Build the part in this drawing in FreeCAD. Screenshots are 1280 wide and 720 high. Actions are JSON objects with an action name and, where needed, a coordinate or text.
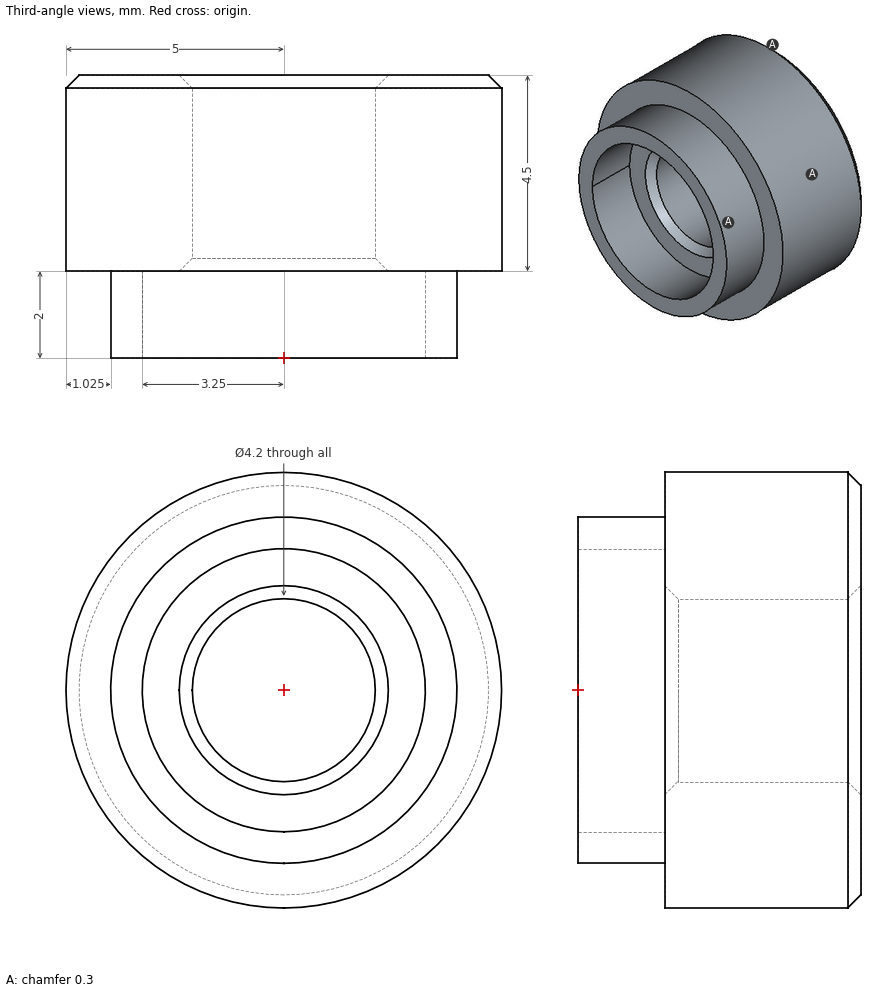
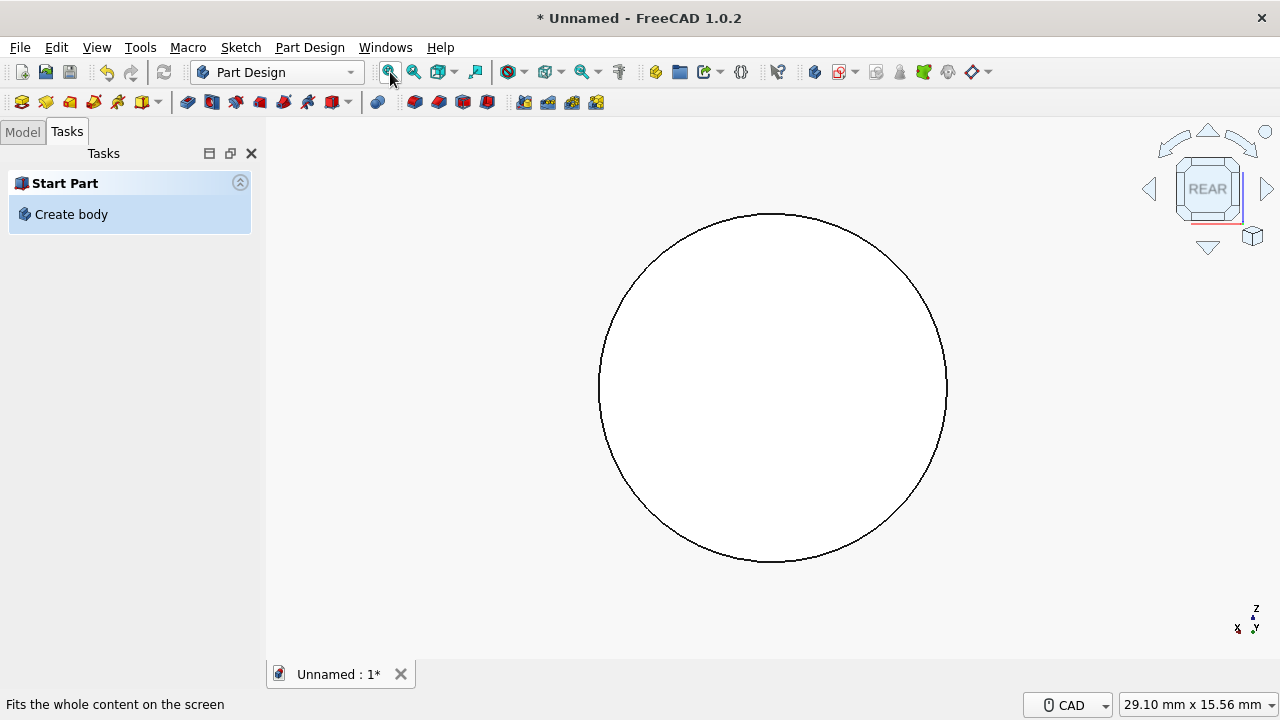
{"action": "left_click", "coordinate": [773, 387]}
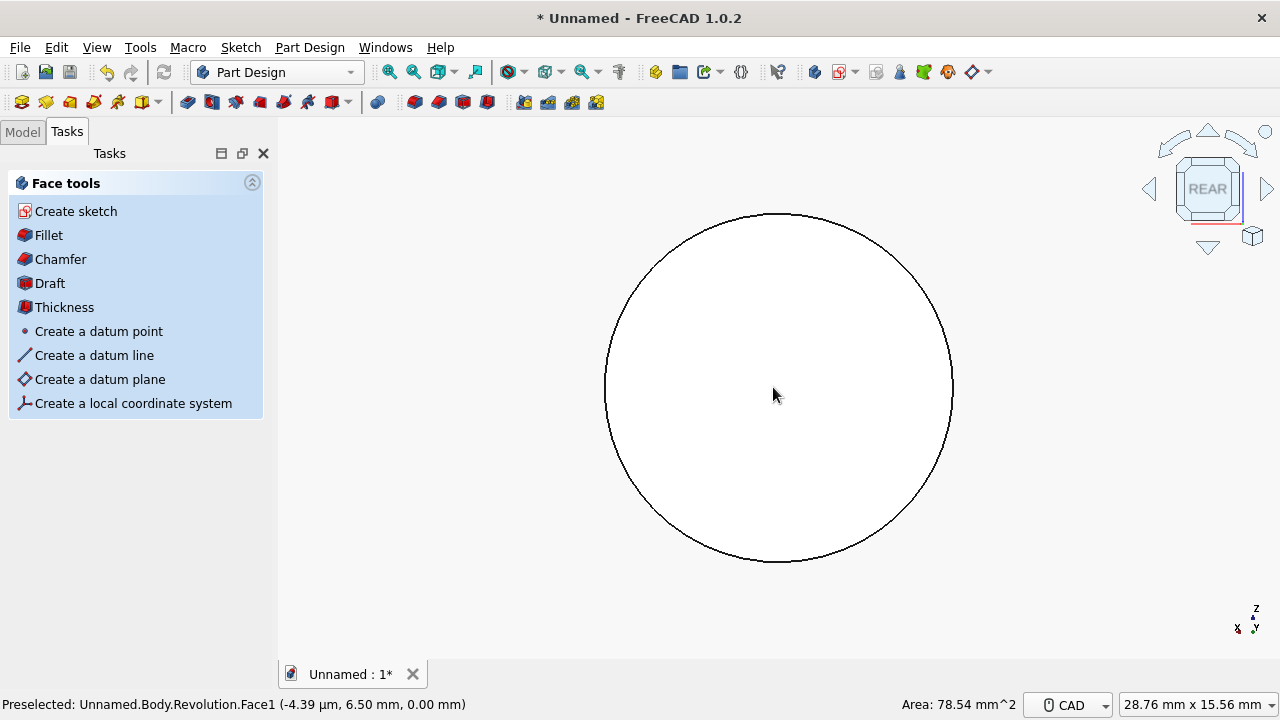
{"action": "left_click", "coordinate": [840, 72]}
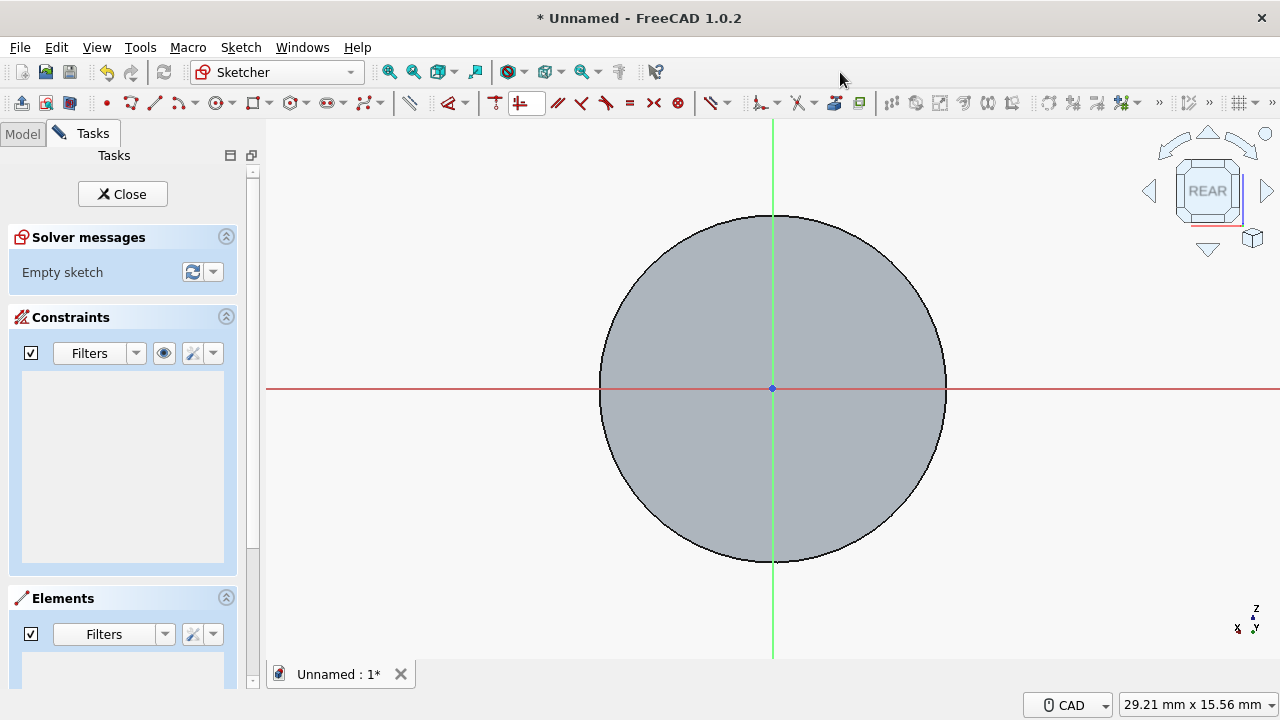
{"action": "scroll", "coordinate": [829, 389], "scroll_direction": "up", "scroll_amount": 4}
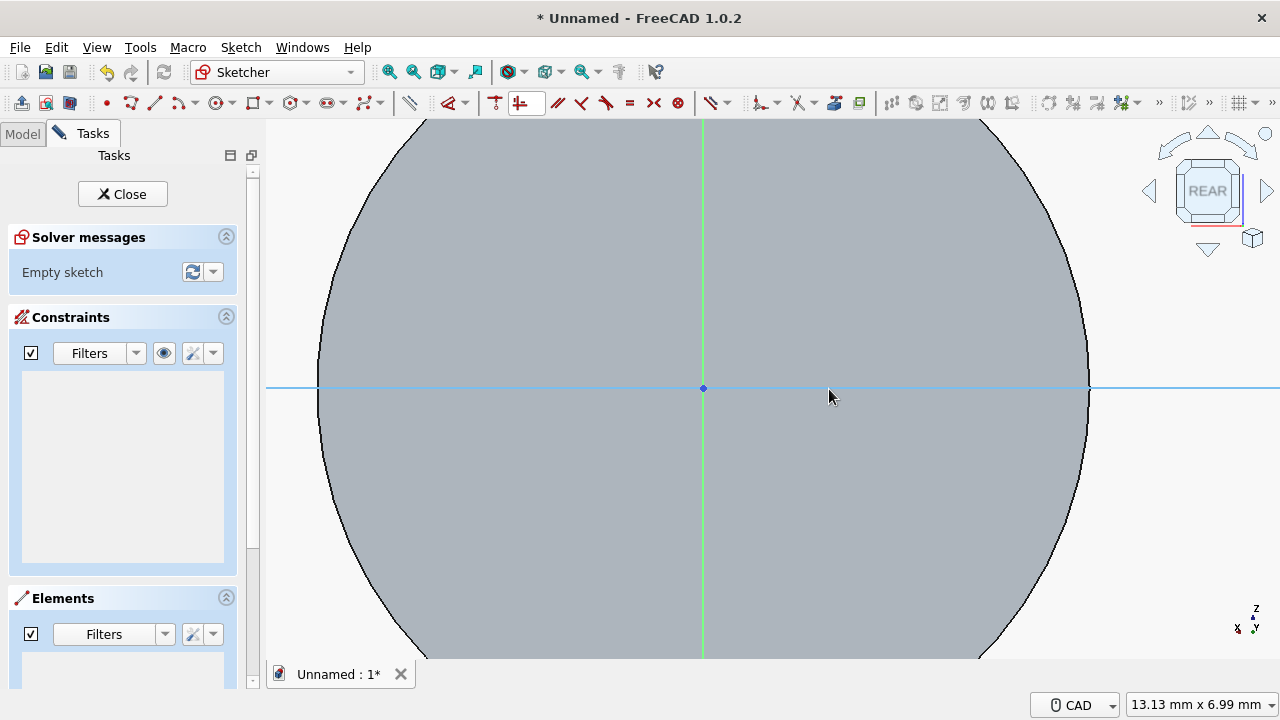
{"action": "left_click", "coordinate": [216, 104]}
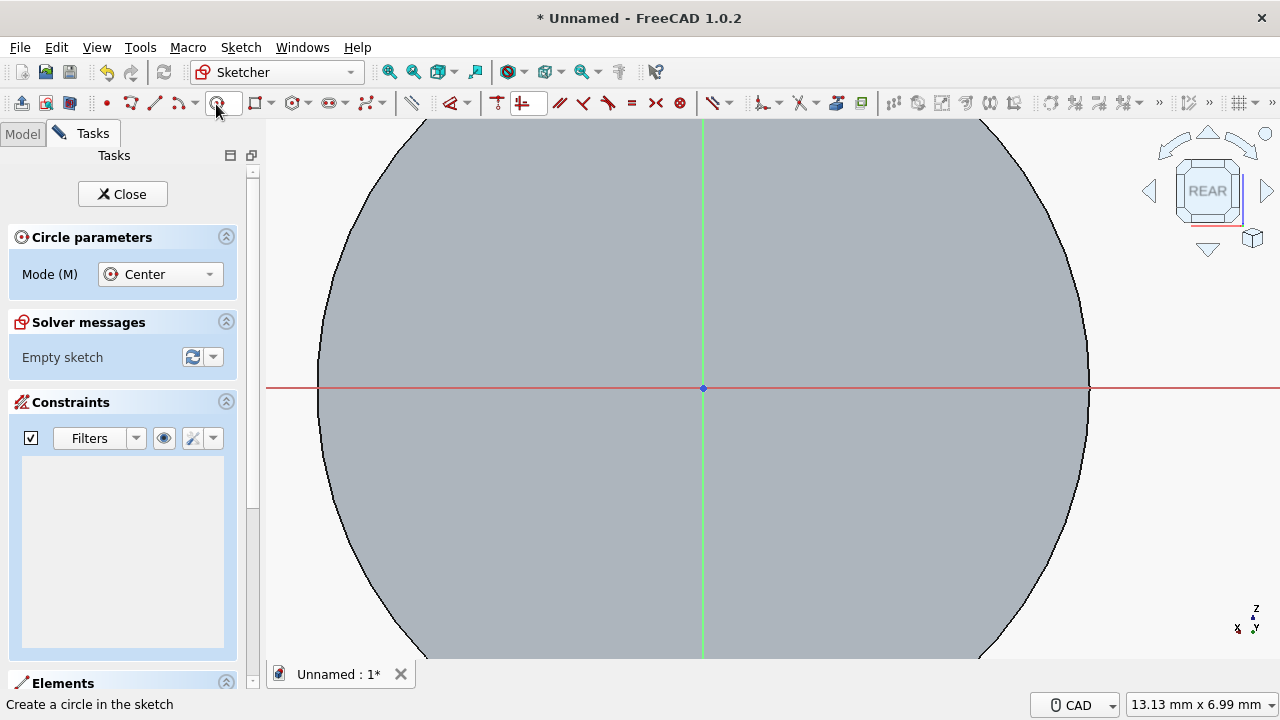
{"action": "left_click", "coordinate": [703, 388]}
{"action": "left_click", "coordinate": [818, 274]}
{"action": "key", "text": "Escape"}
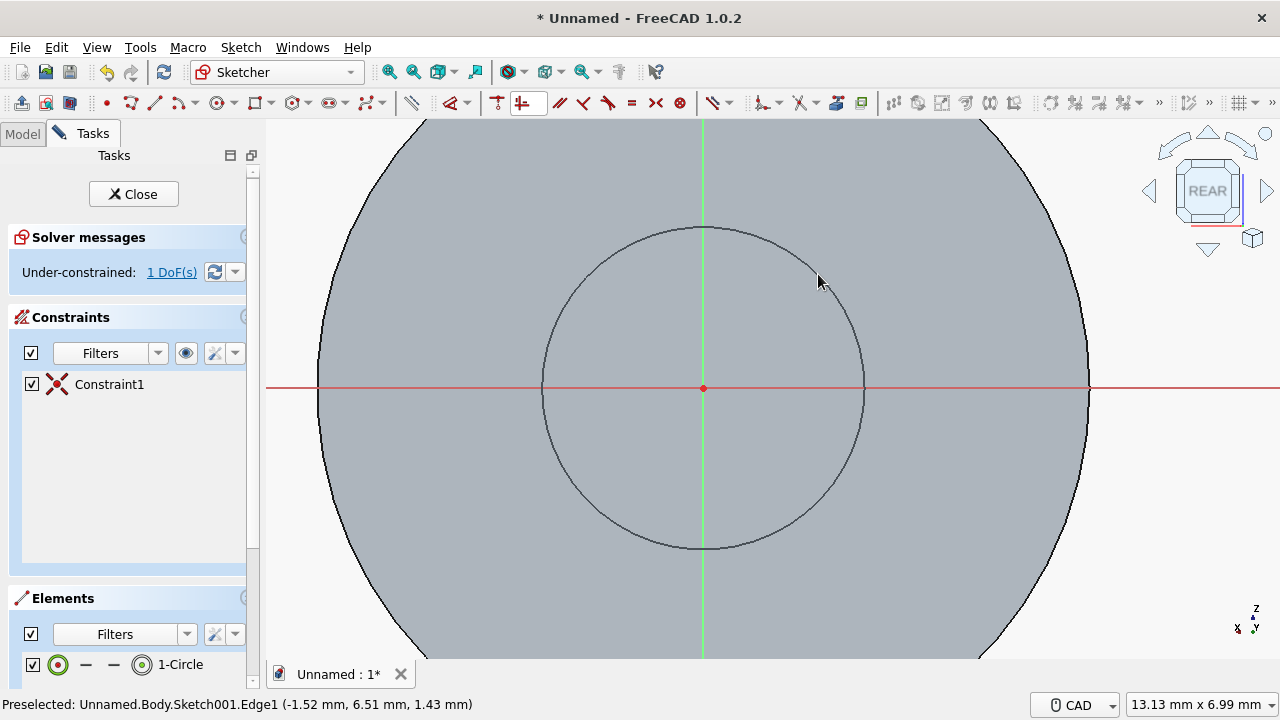
{"action": "left_click", "coordinate": [450, 104]}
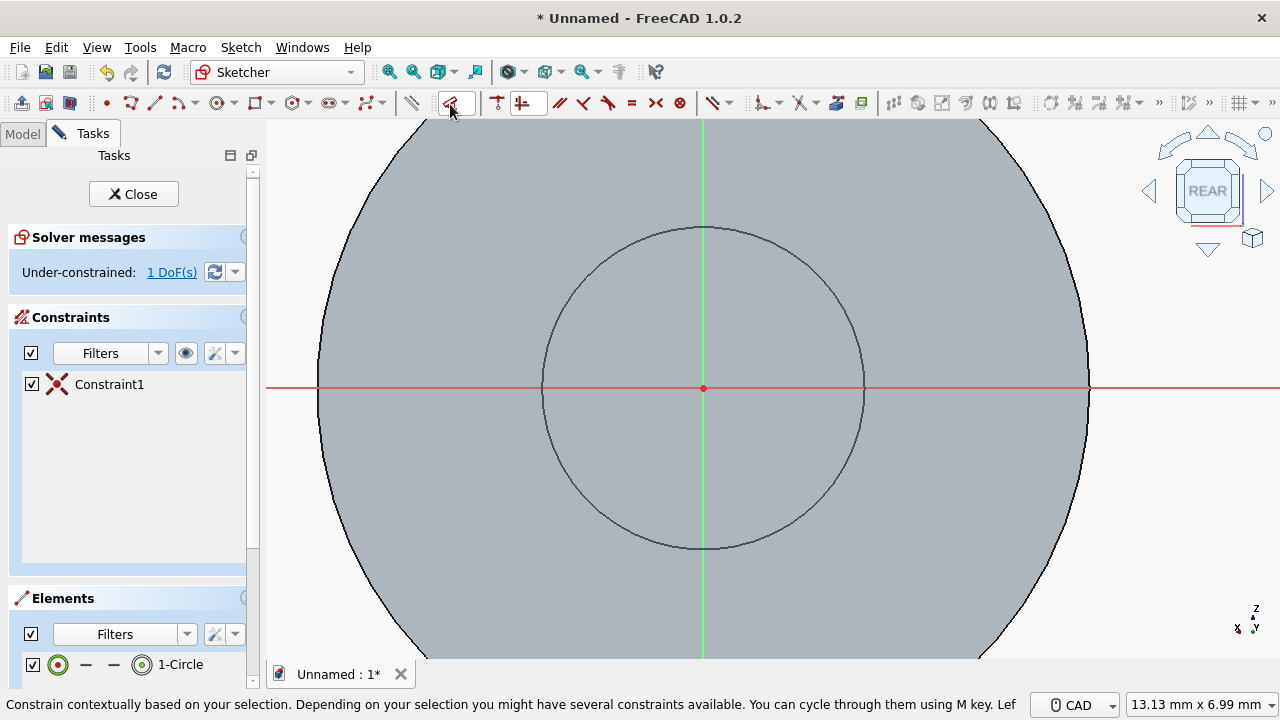
{"action": "left_click", "coordinate": [817, 274]}
{"action": "left_click", "coordinate": [840, 251]}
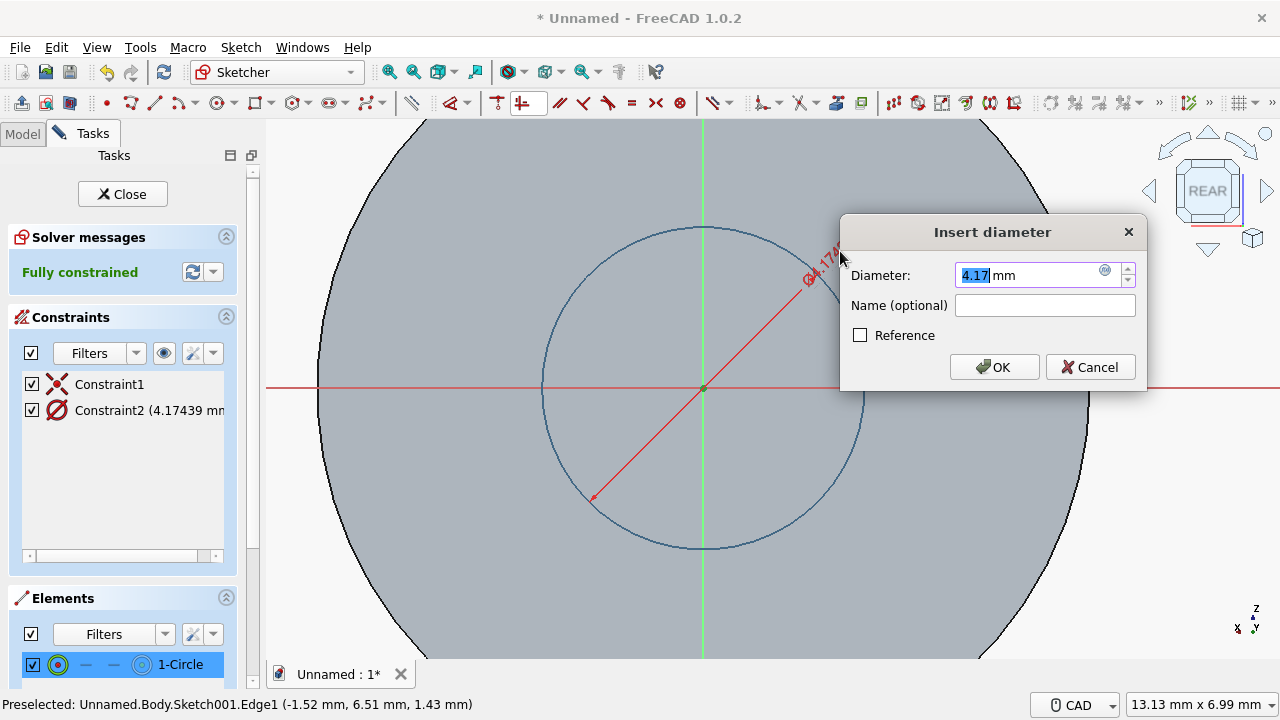
{"action": "type", "text": "4.2"}
{"action": "key", "text": "Return"}
{"action": "key", "text": "Escape"}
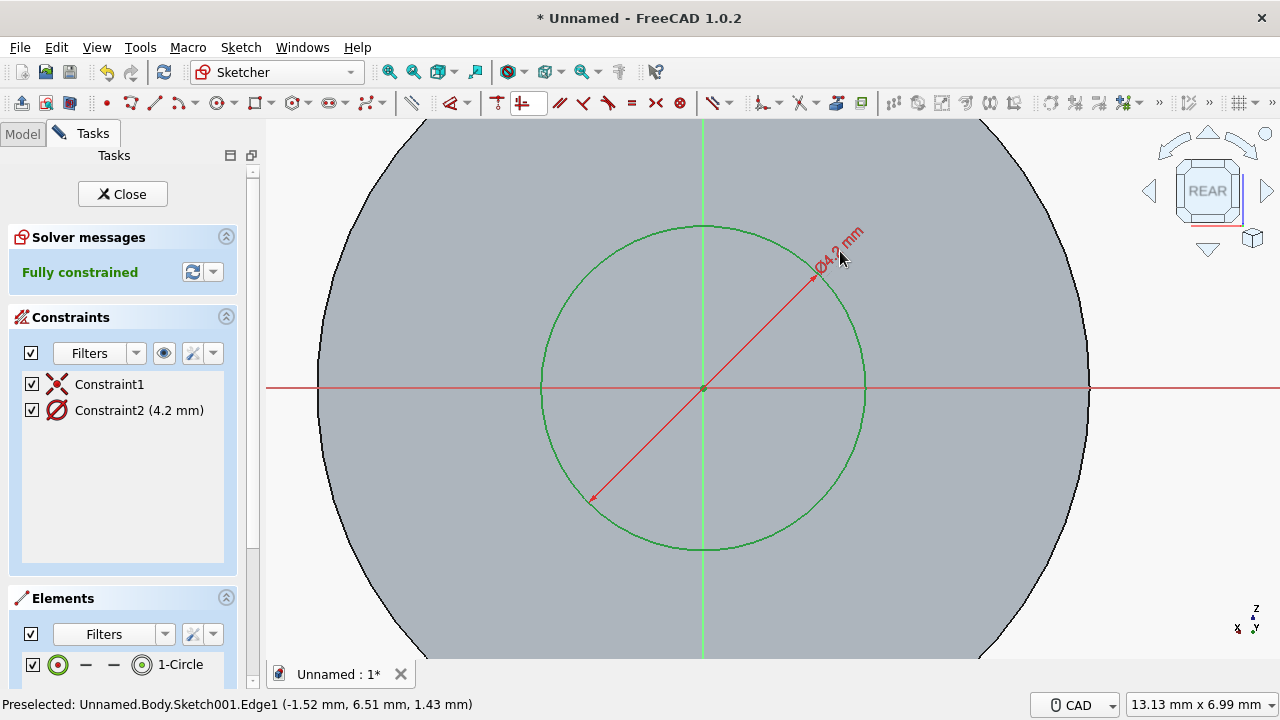
{"action": "left_click", "coordinate": [123, 194]}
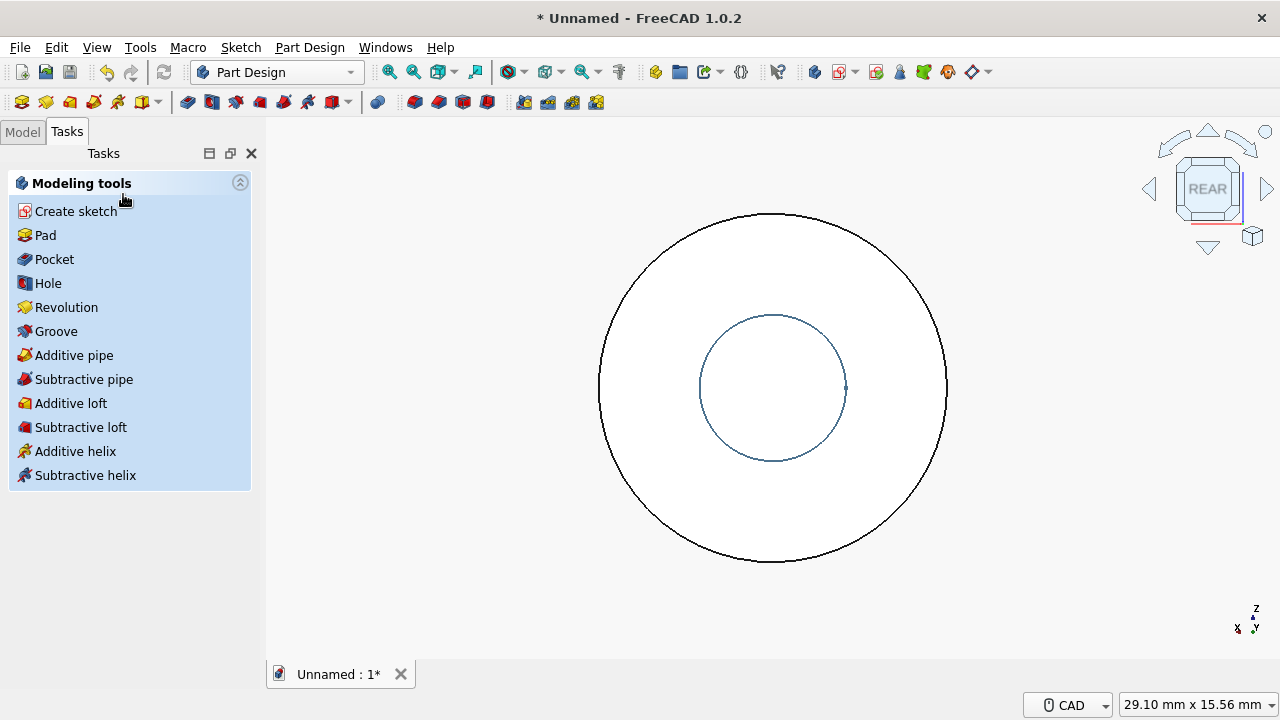
{"action": "left_click", "coordinate": [212, 102]}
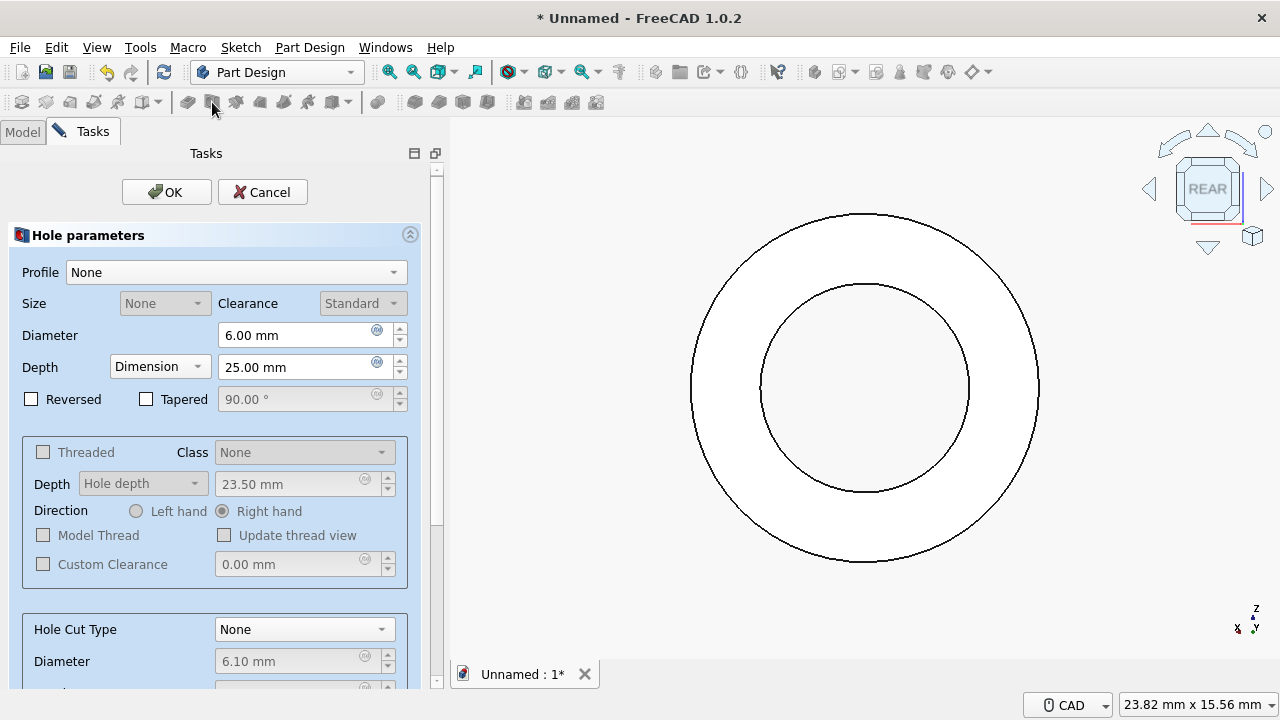
{"action": "triple_click", "coordinate": [305, 335]}